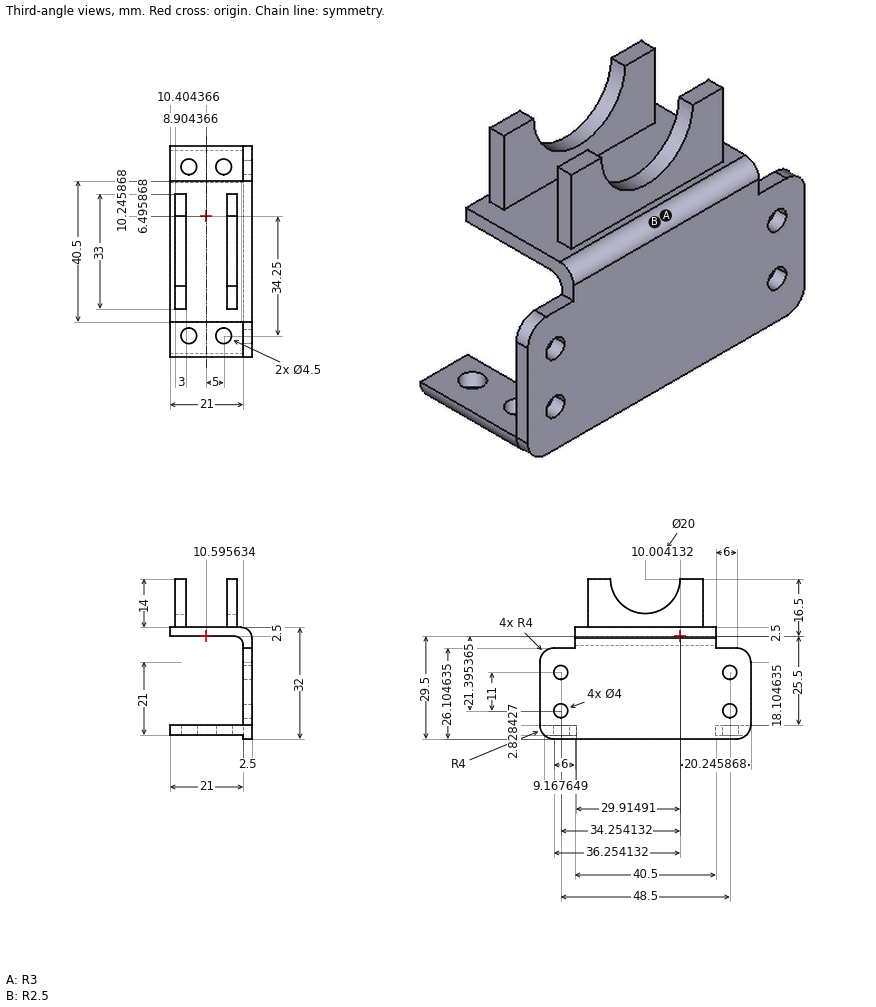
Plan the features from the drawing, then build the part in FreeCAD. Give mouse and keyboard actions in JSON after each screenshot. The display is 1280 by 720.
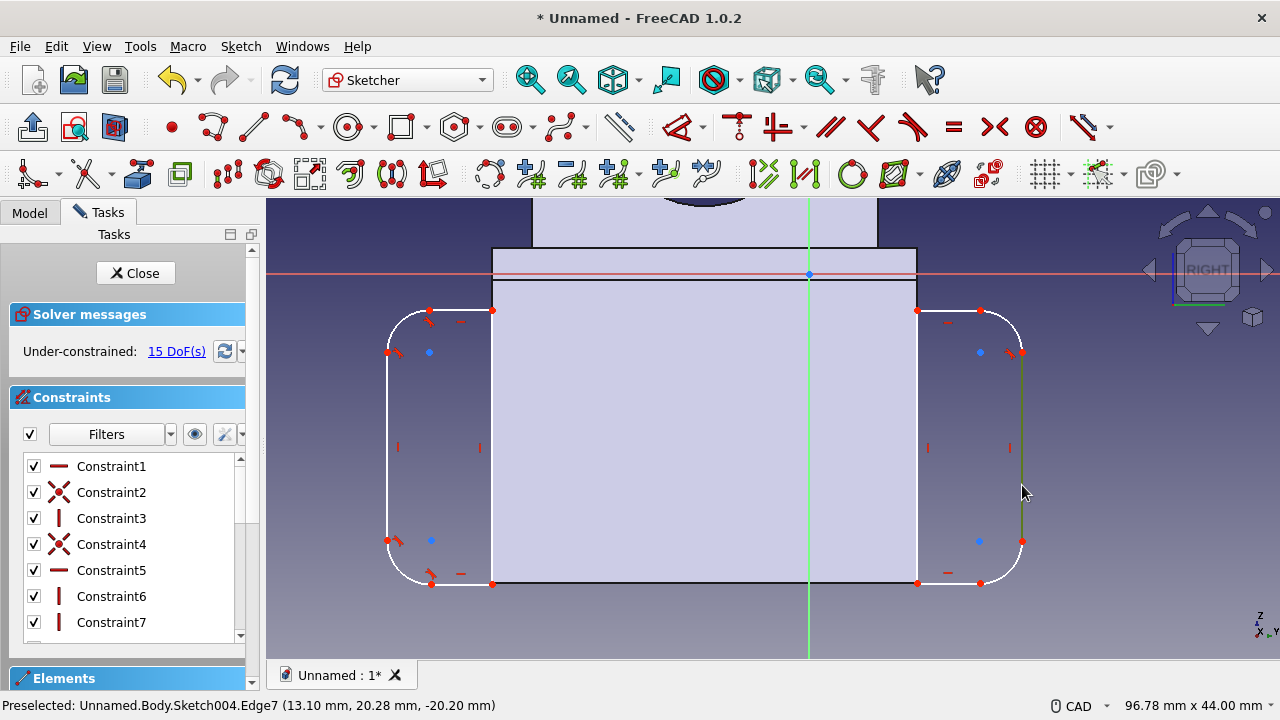
{"action": "left_click", "coordinate": [999, 579]}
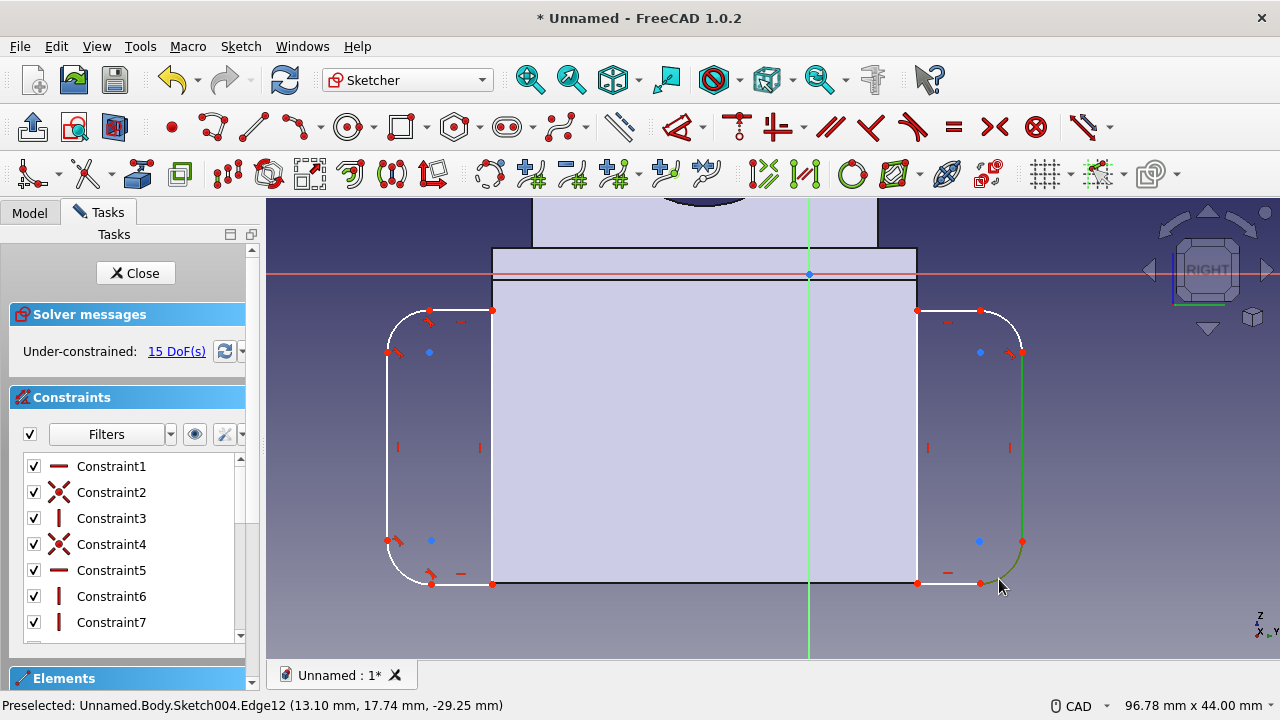
{"action": "left_click", "coordinate": [913, 128]}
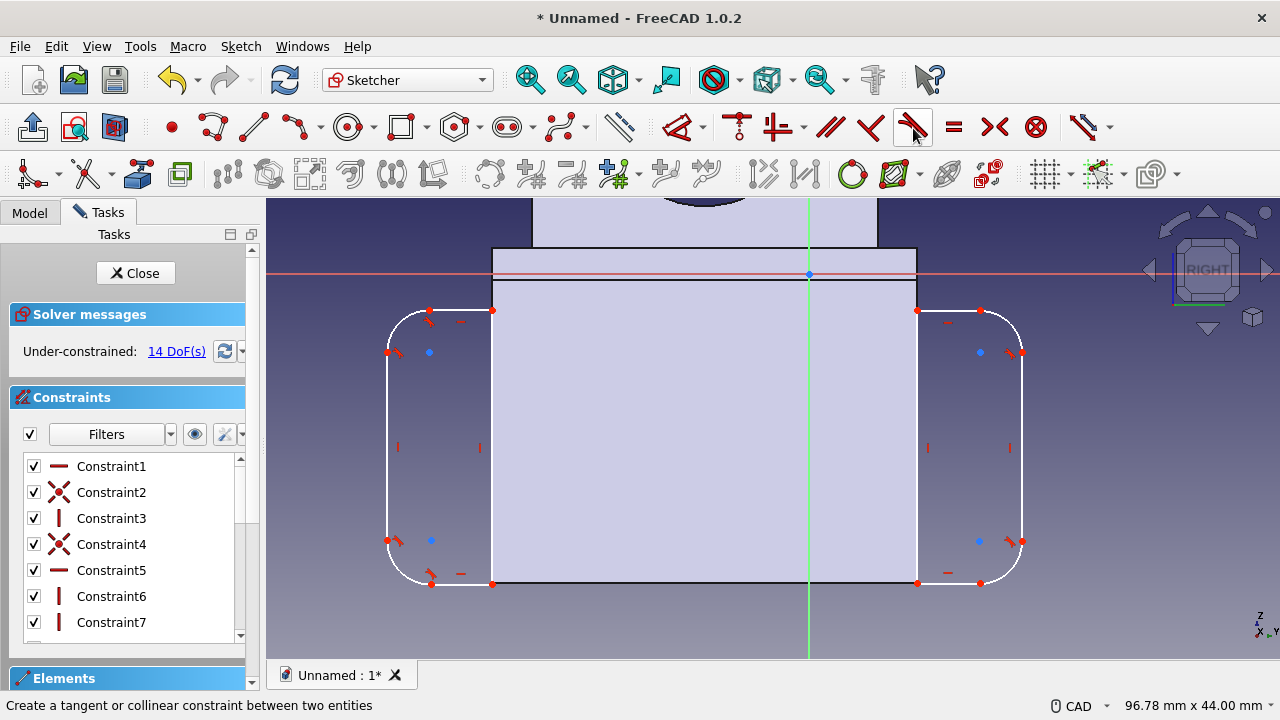
{"action": "left_click", "coordinate": [961, 311]}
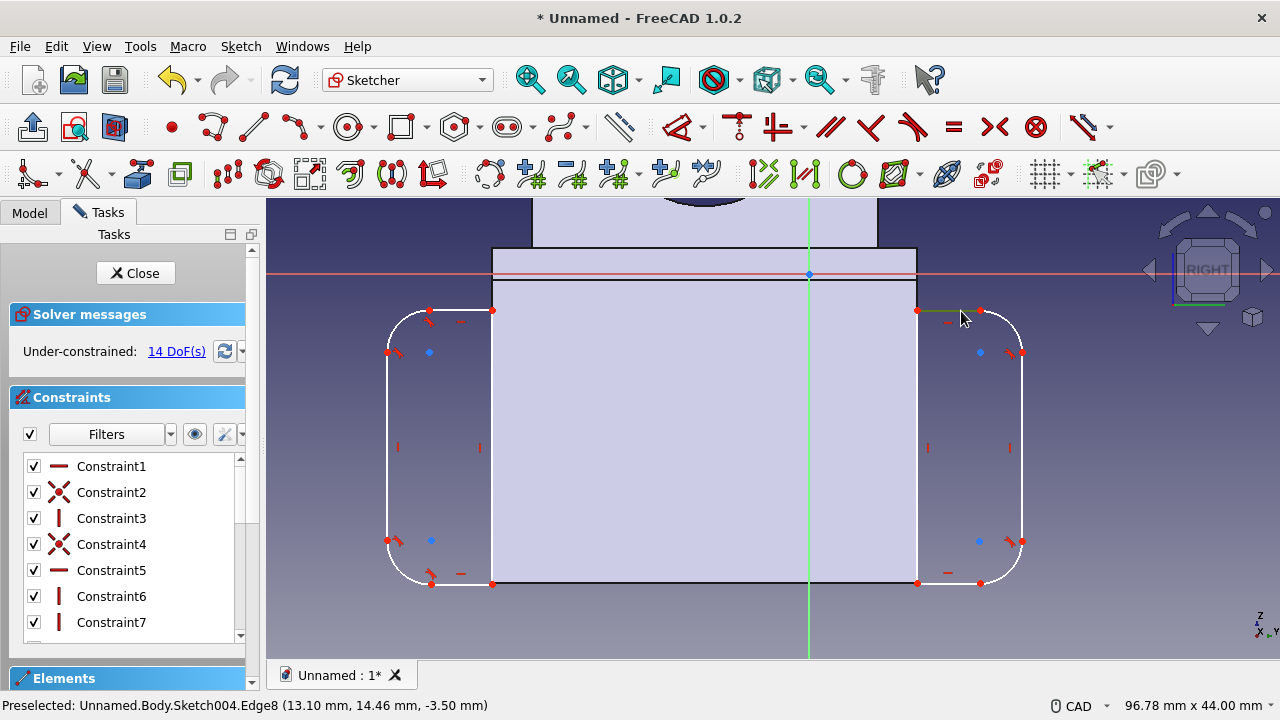
{"action": "left_click", "coordinate": [1017, 334]}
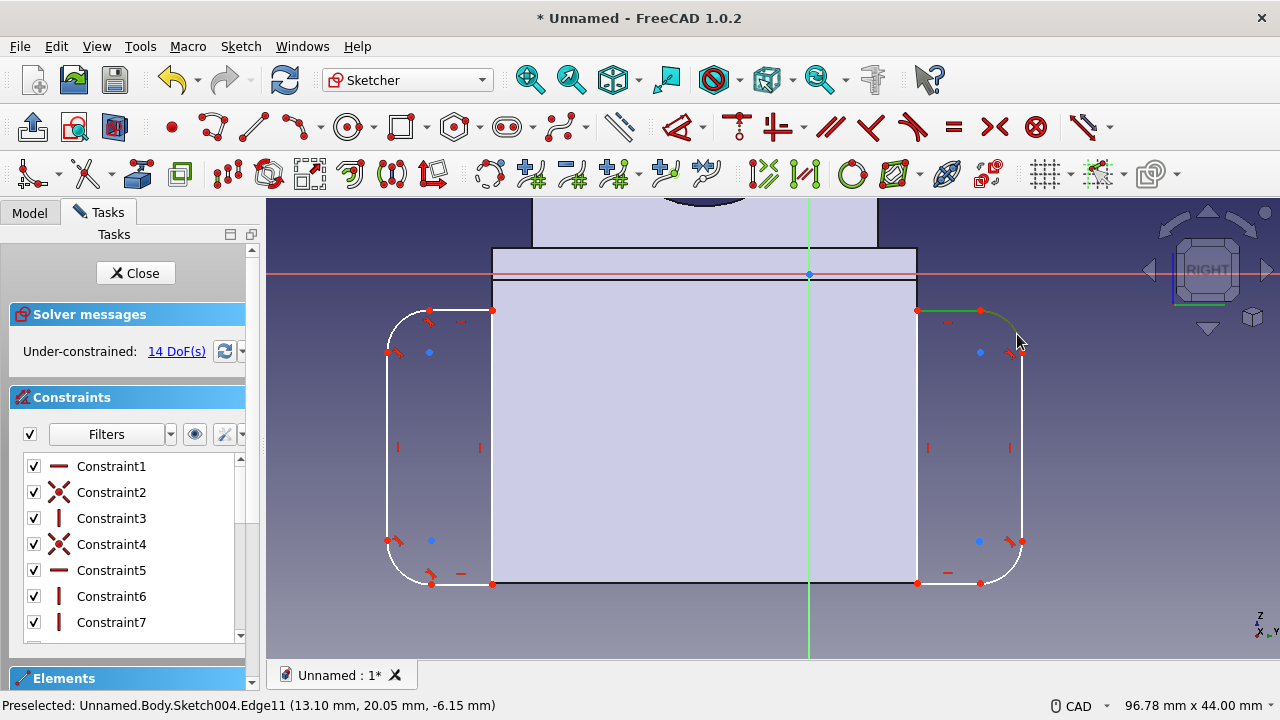
{"action": "left_click", "coordinate": [913, 128]}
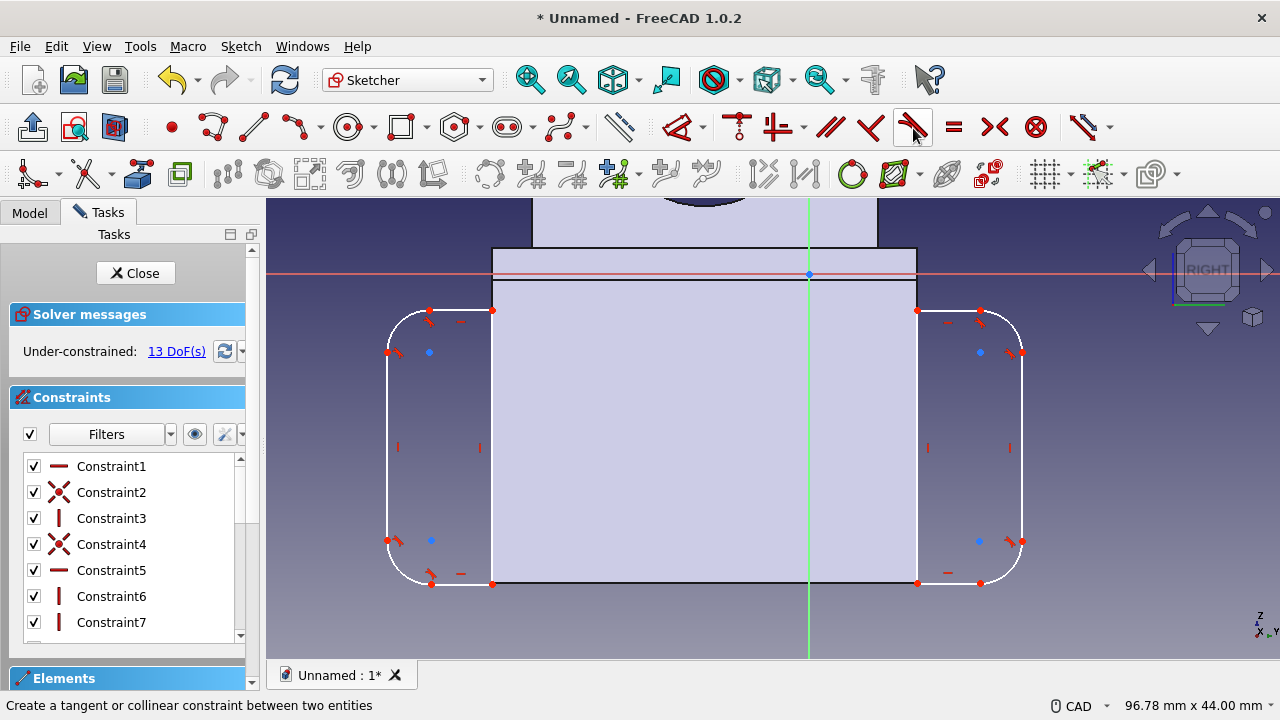
{"action": "left_click", "coordinate": [936, 584]}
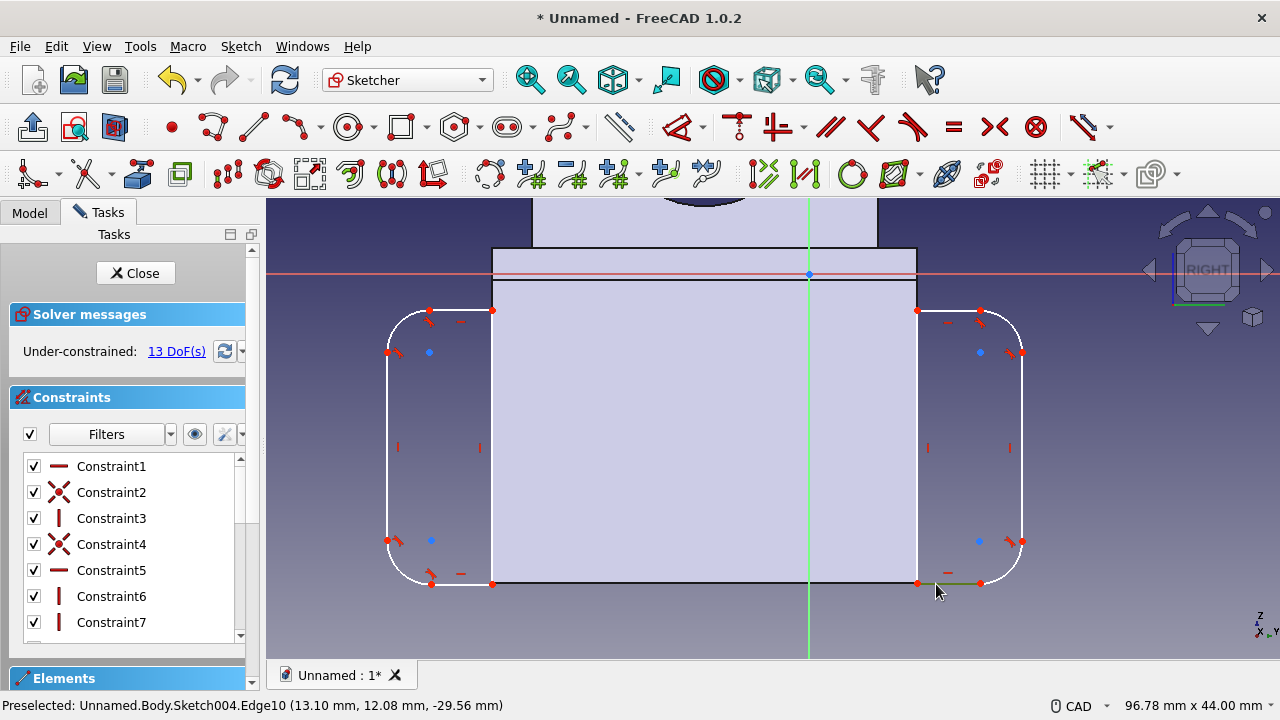
{"action": "left_click", "coordinate": [999, 579]}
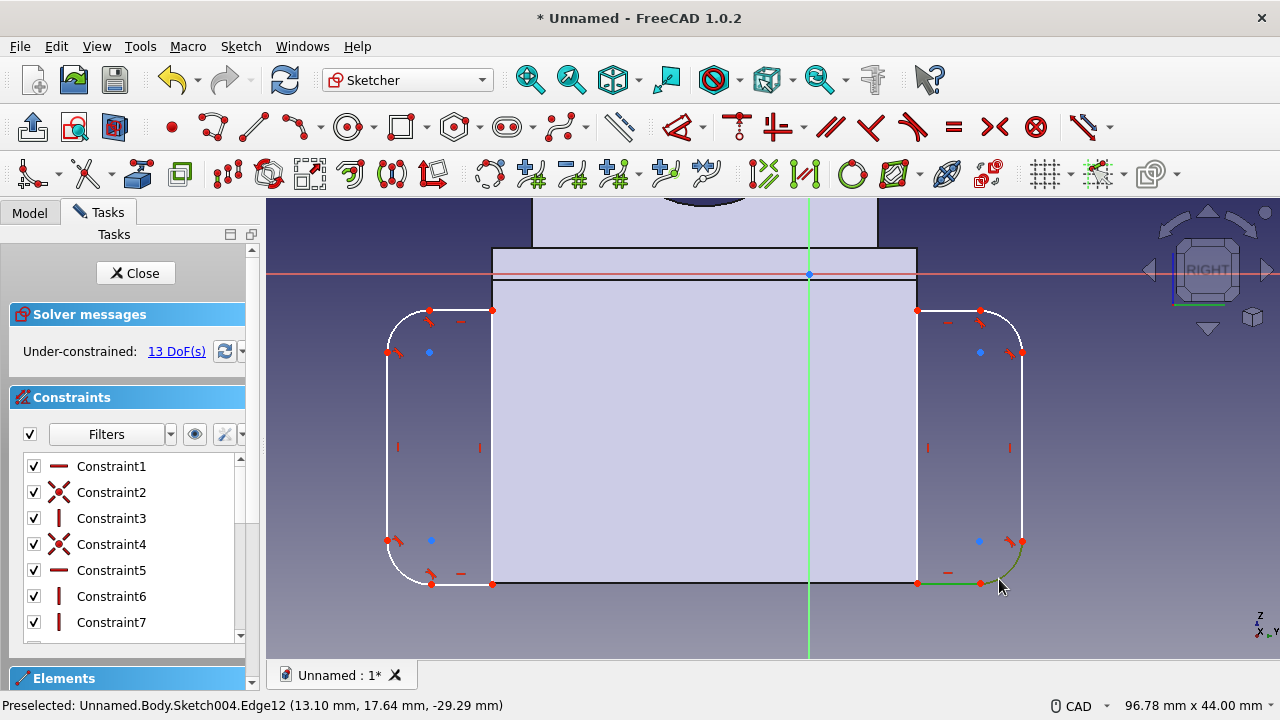
{"action": "left_click", "coordinate": [913, 128]}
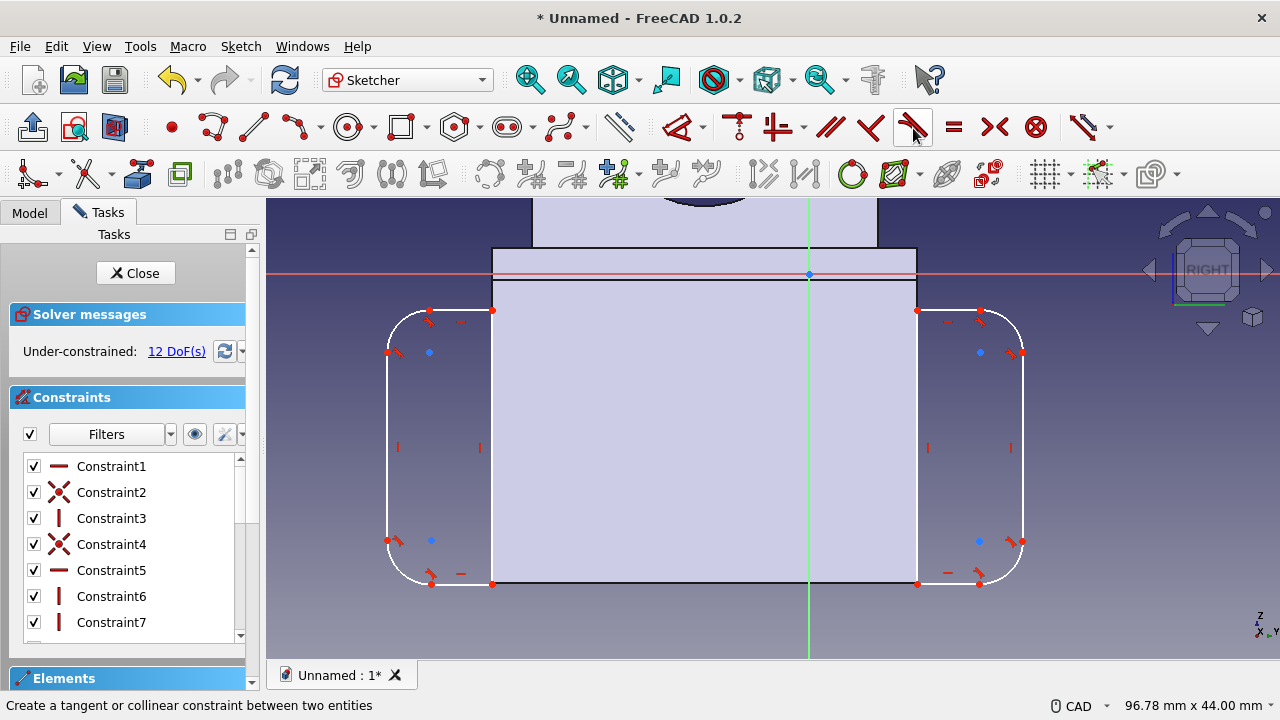
{"action": "left_click", "coordinate": [410, 315]}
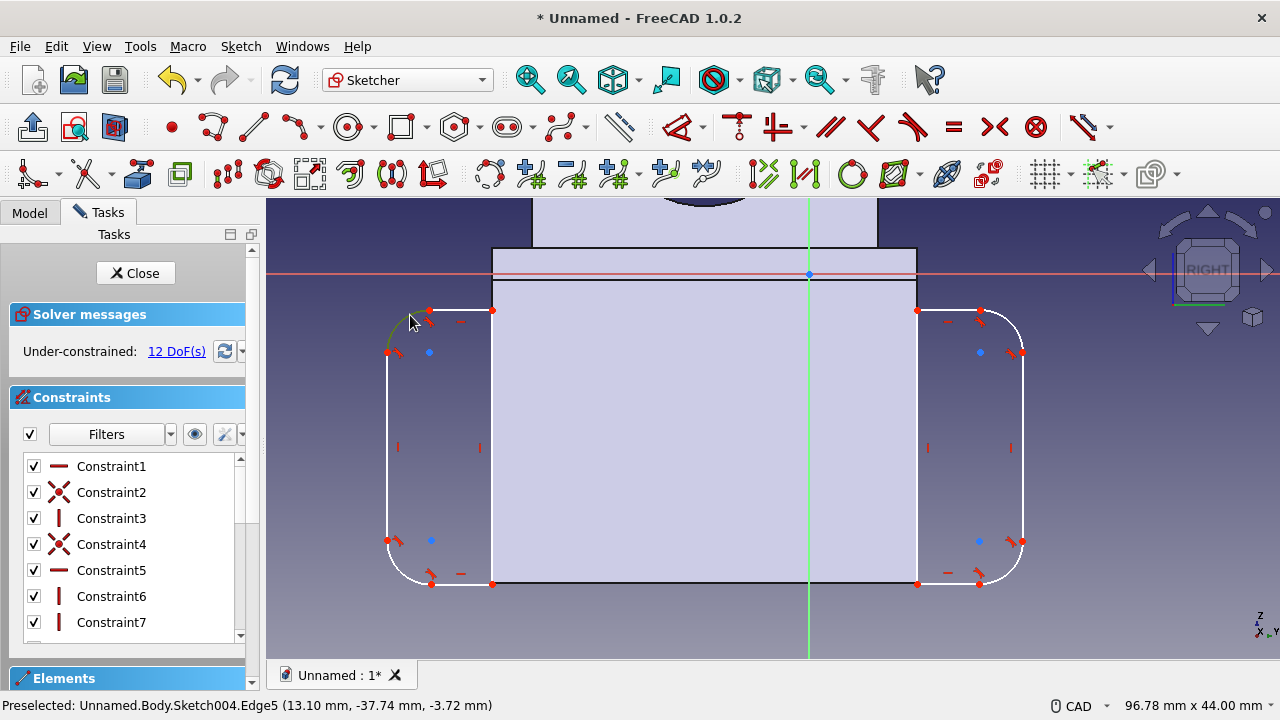
{"action": "left_click", "coordinate": [392, 561]}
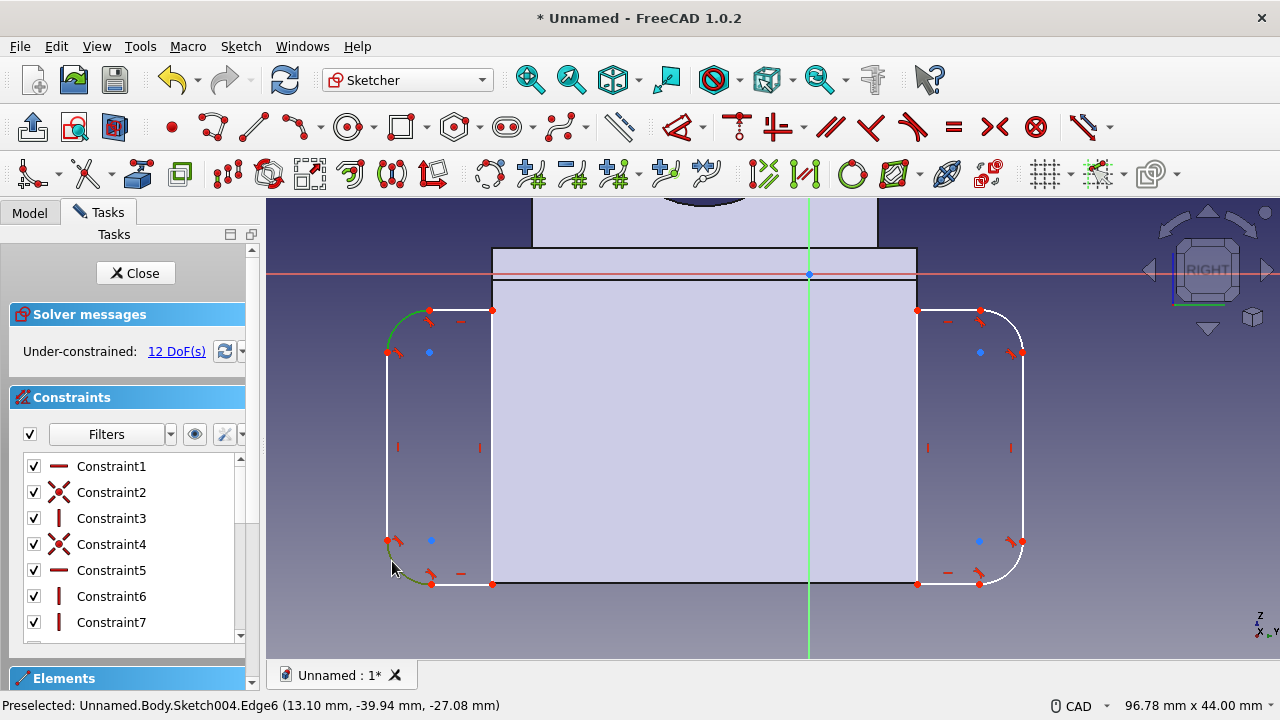
{"action": "left_click", "coordinate": [1018, 333]}